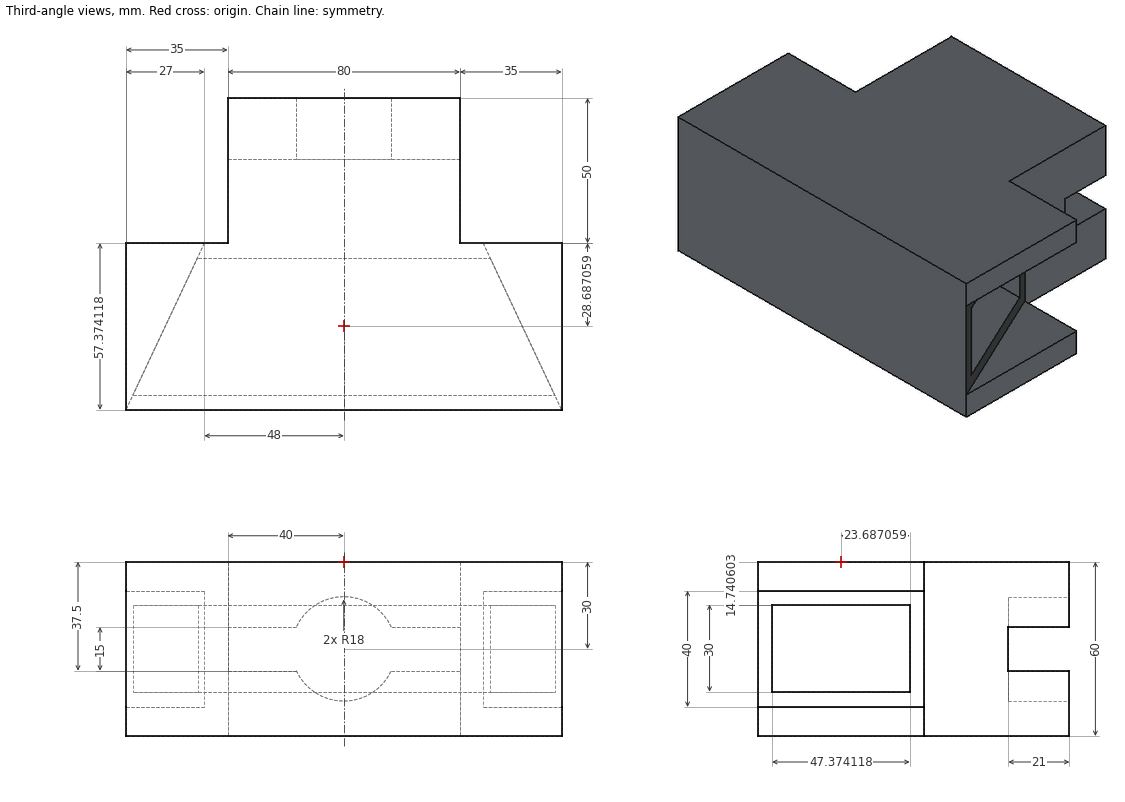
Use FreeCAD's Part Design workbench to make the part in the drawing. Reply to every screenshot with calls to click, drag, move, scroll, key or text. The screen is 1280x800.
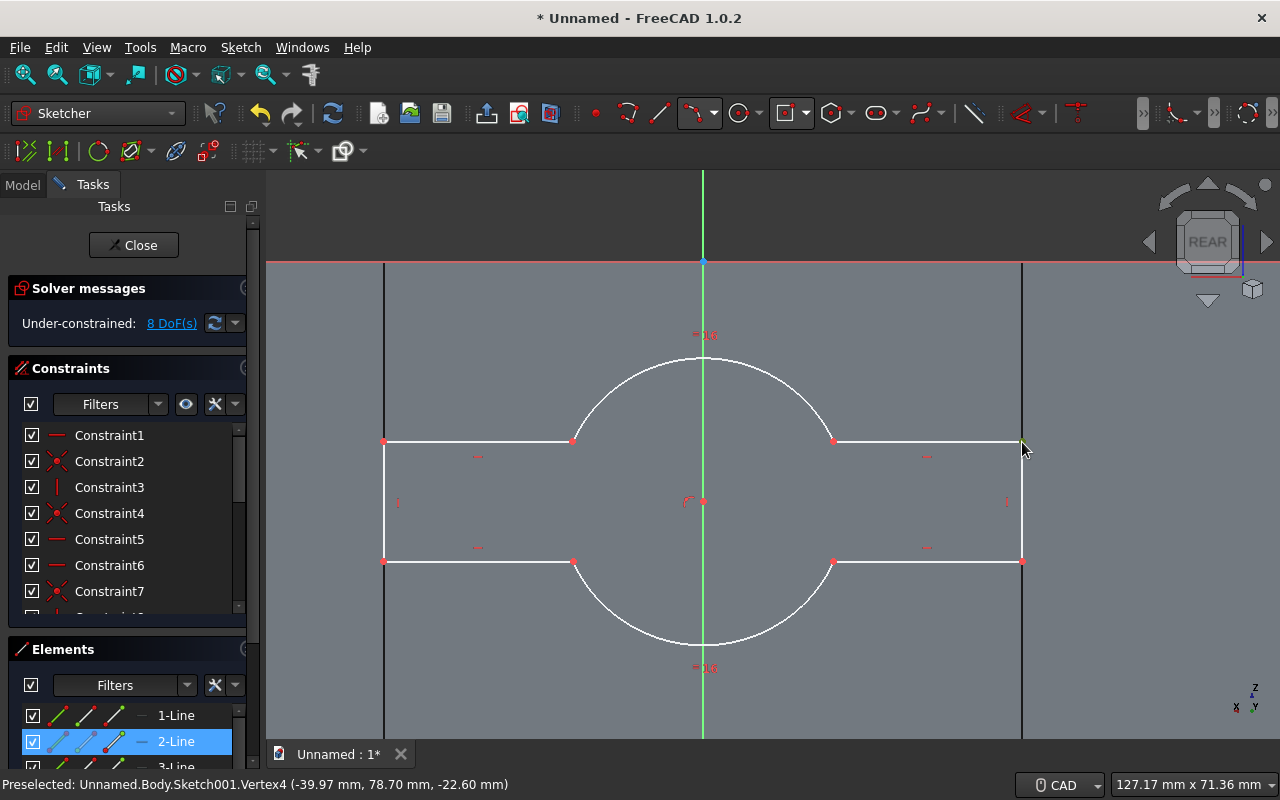
click(384, 442)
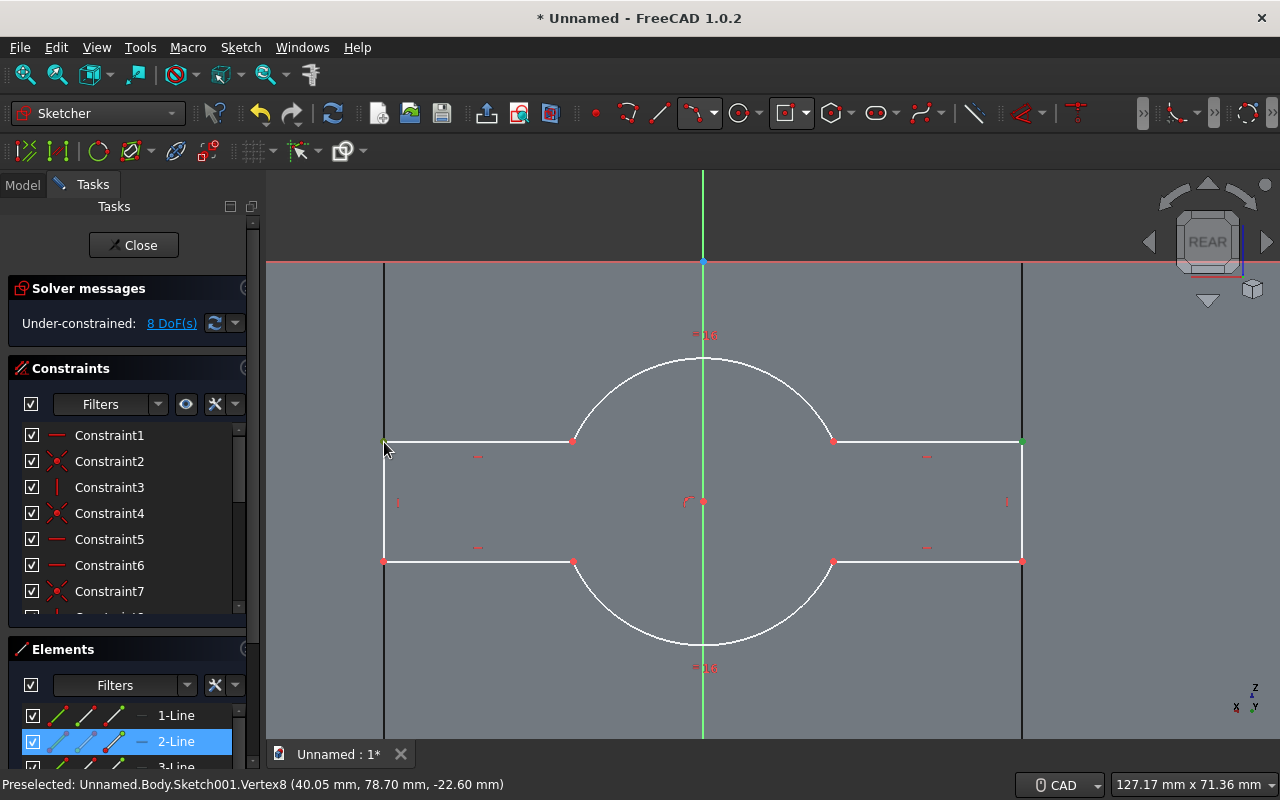
click(703, 601)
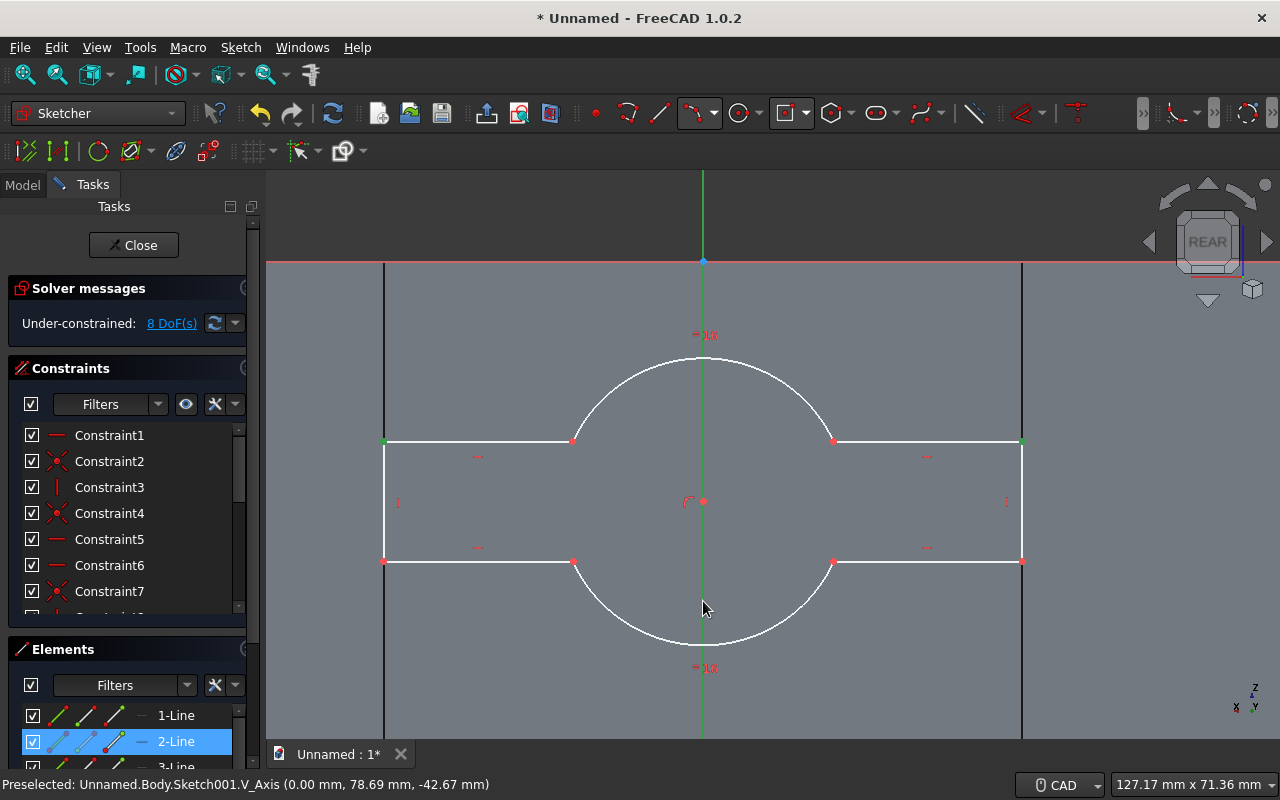
key(s)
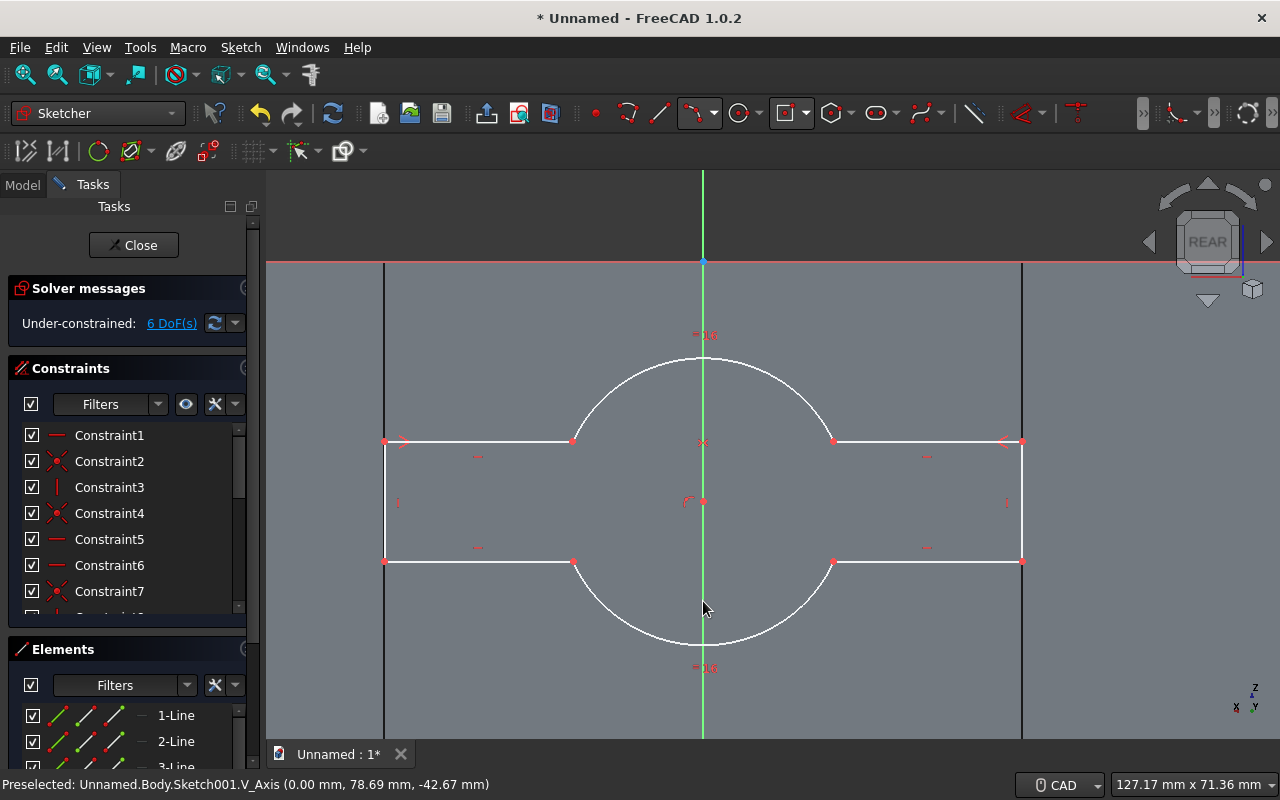
key(d)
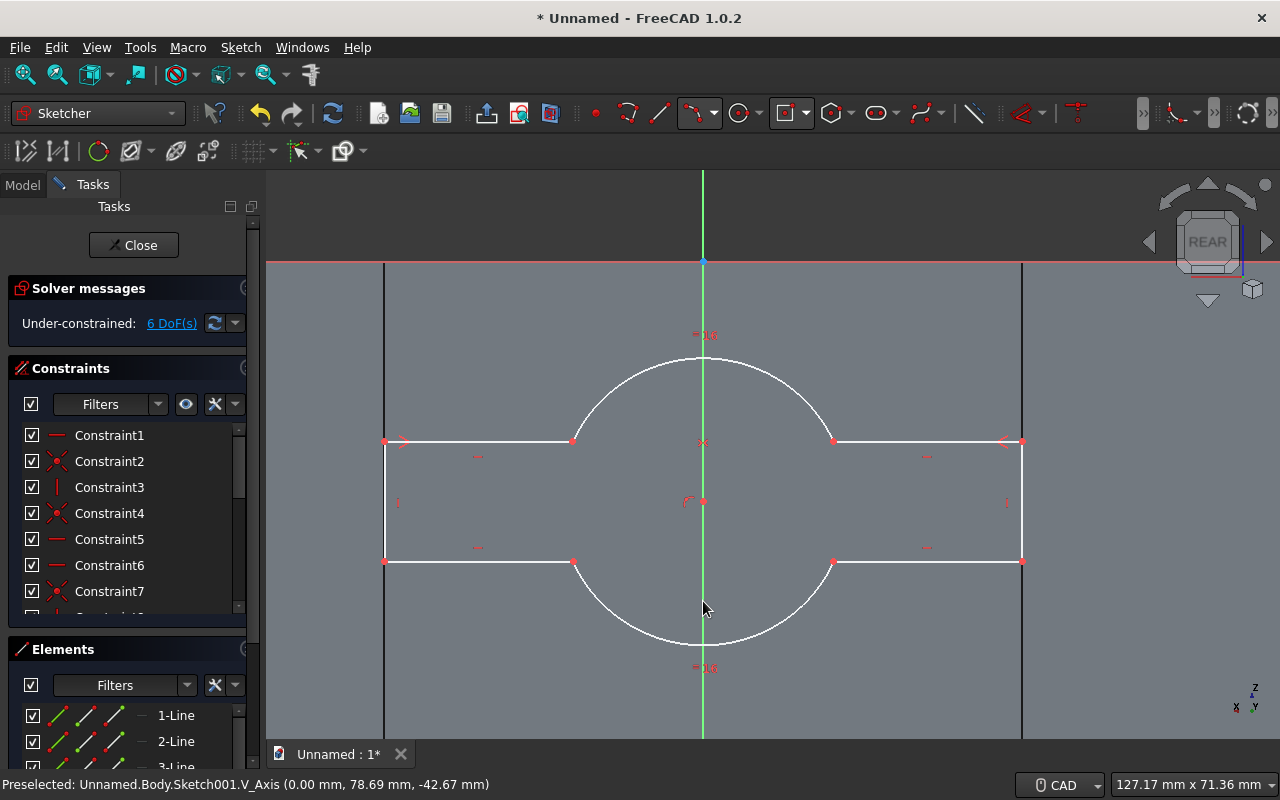
click(767, 373)
click(781, 344)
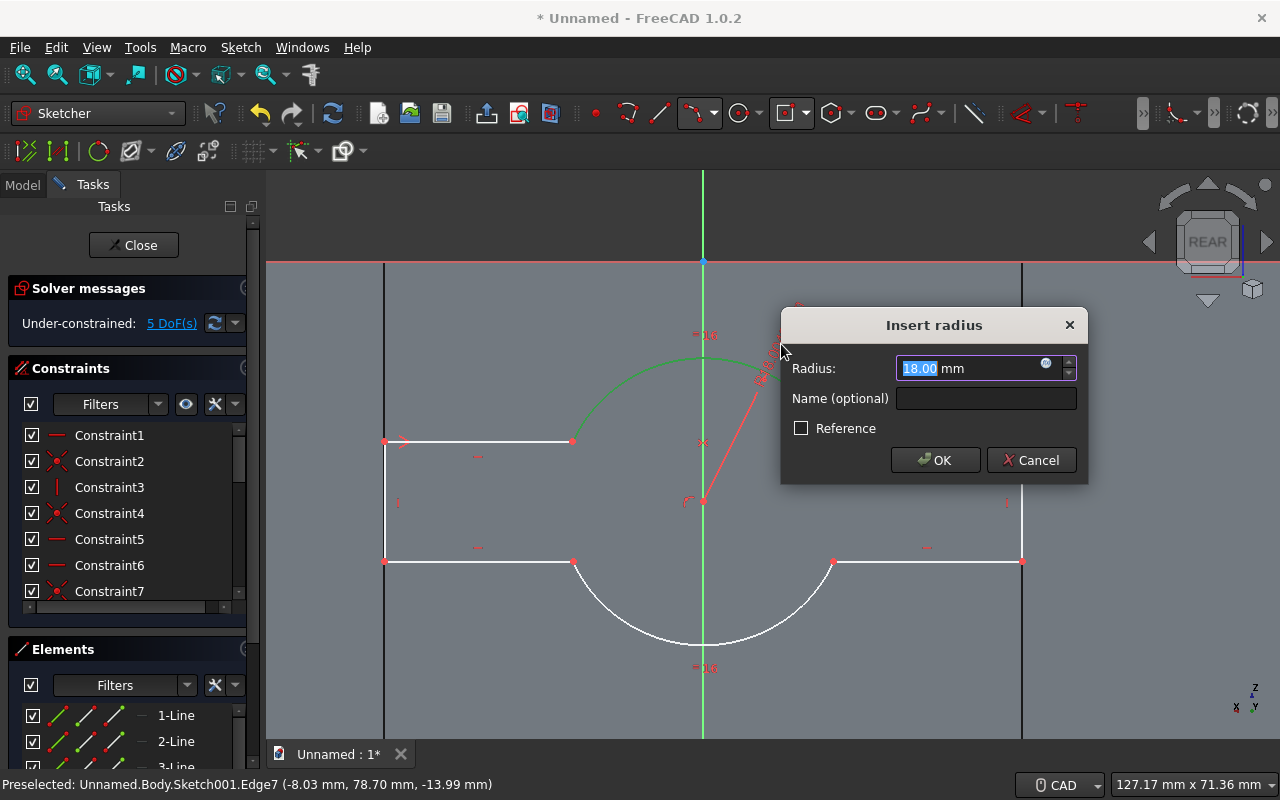
text(18)
key(Return)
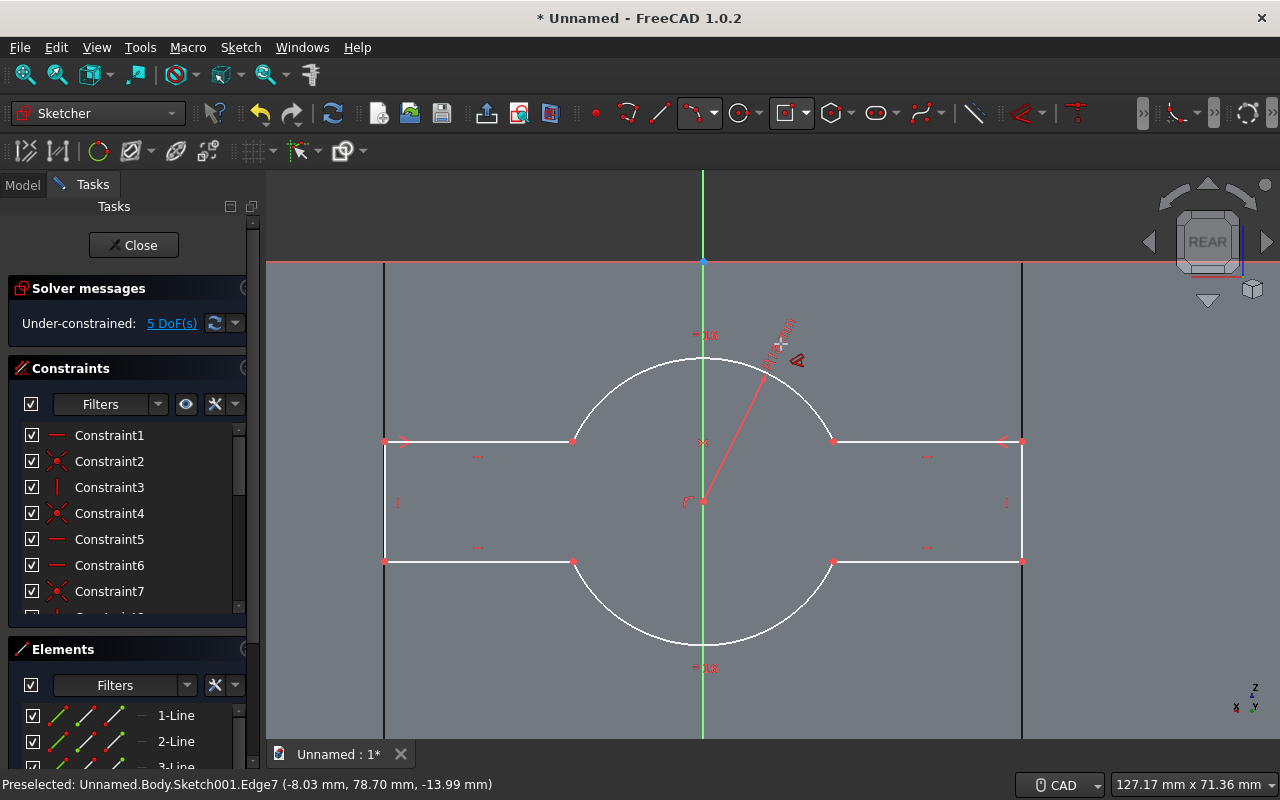
click(1022, 526)
click(1056, 502)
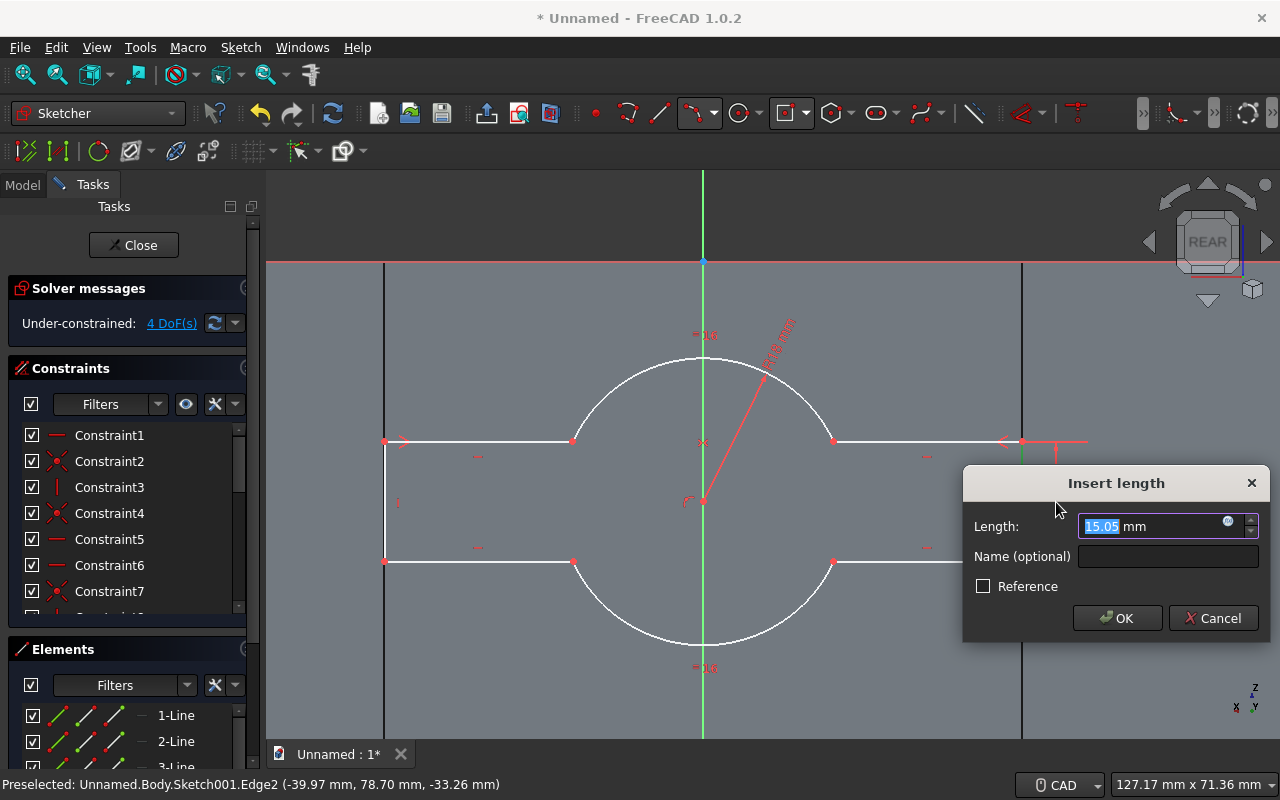
text(15)
key(Return)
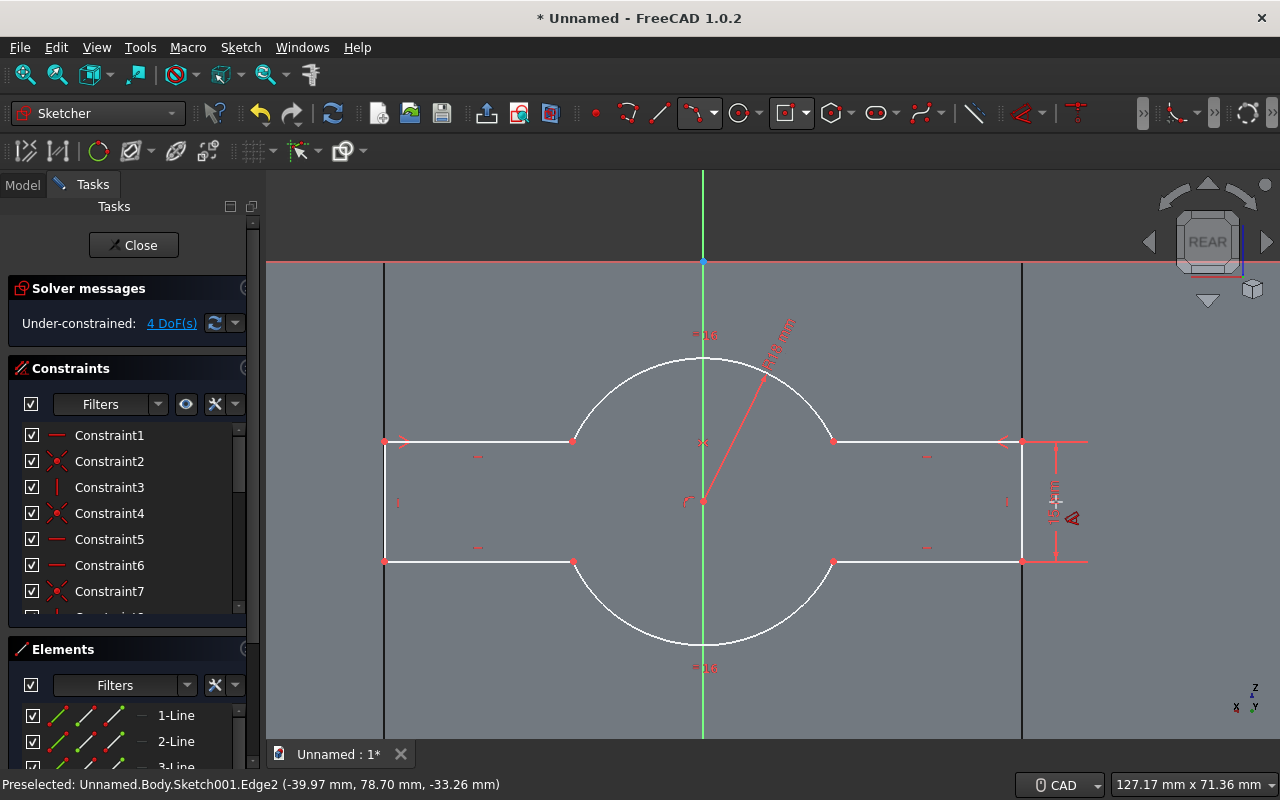
click(385, 478)
click(351, 502)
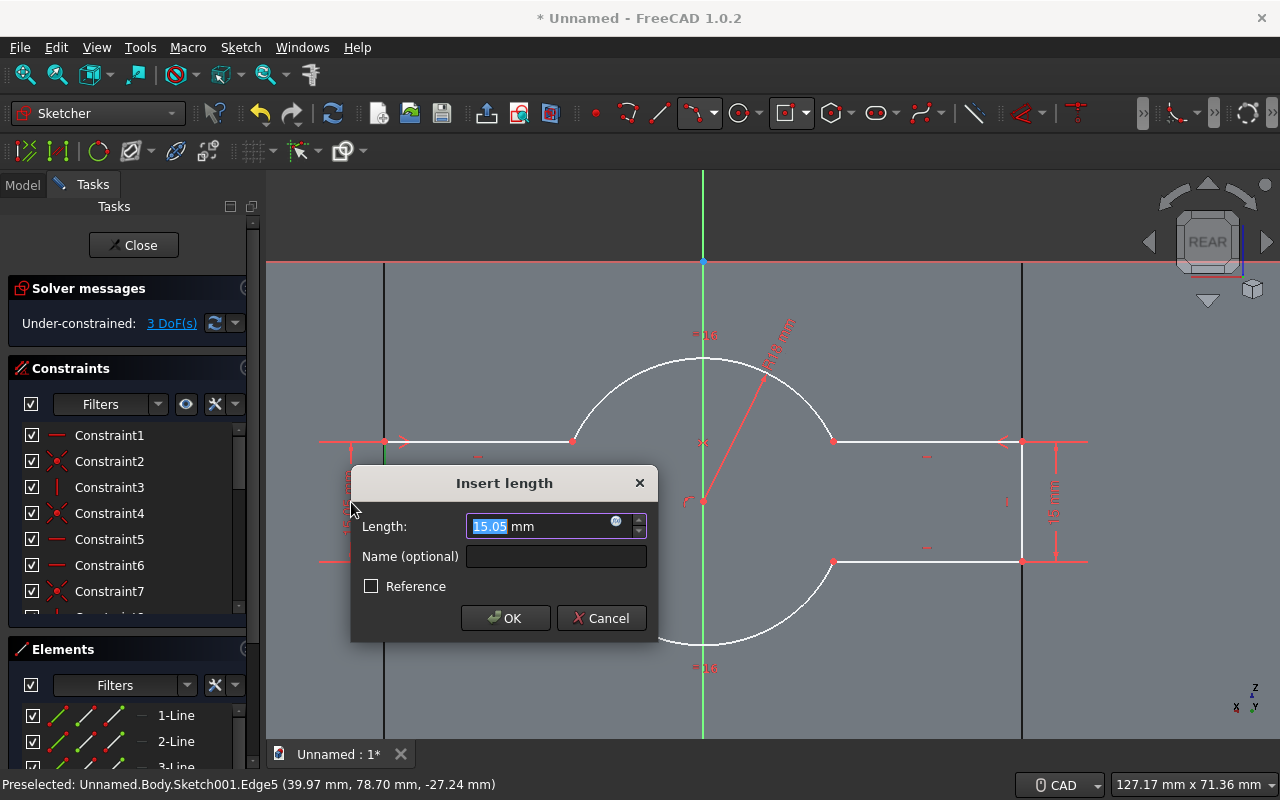
text(15)
key(Return)